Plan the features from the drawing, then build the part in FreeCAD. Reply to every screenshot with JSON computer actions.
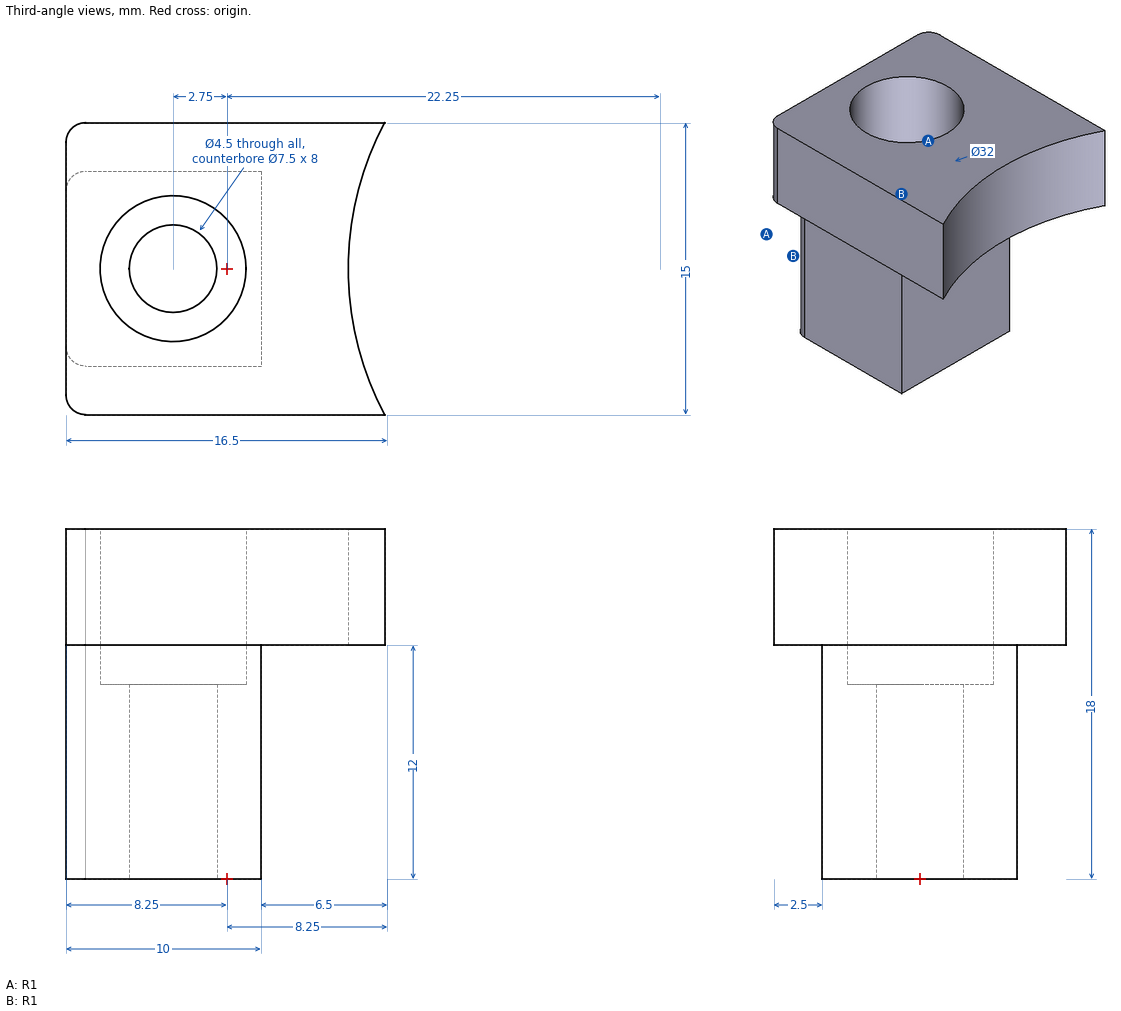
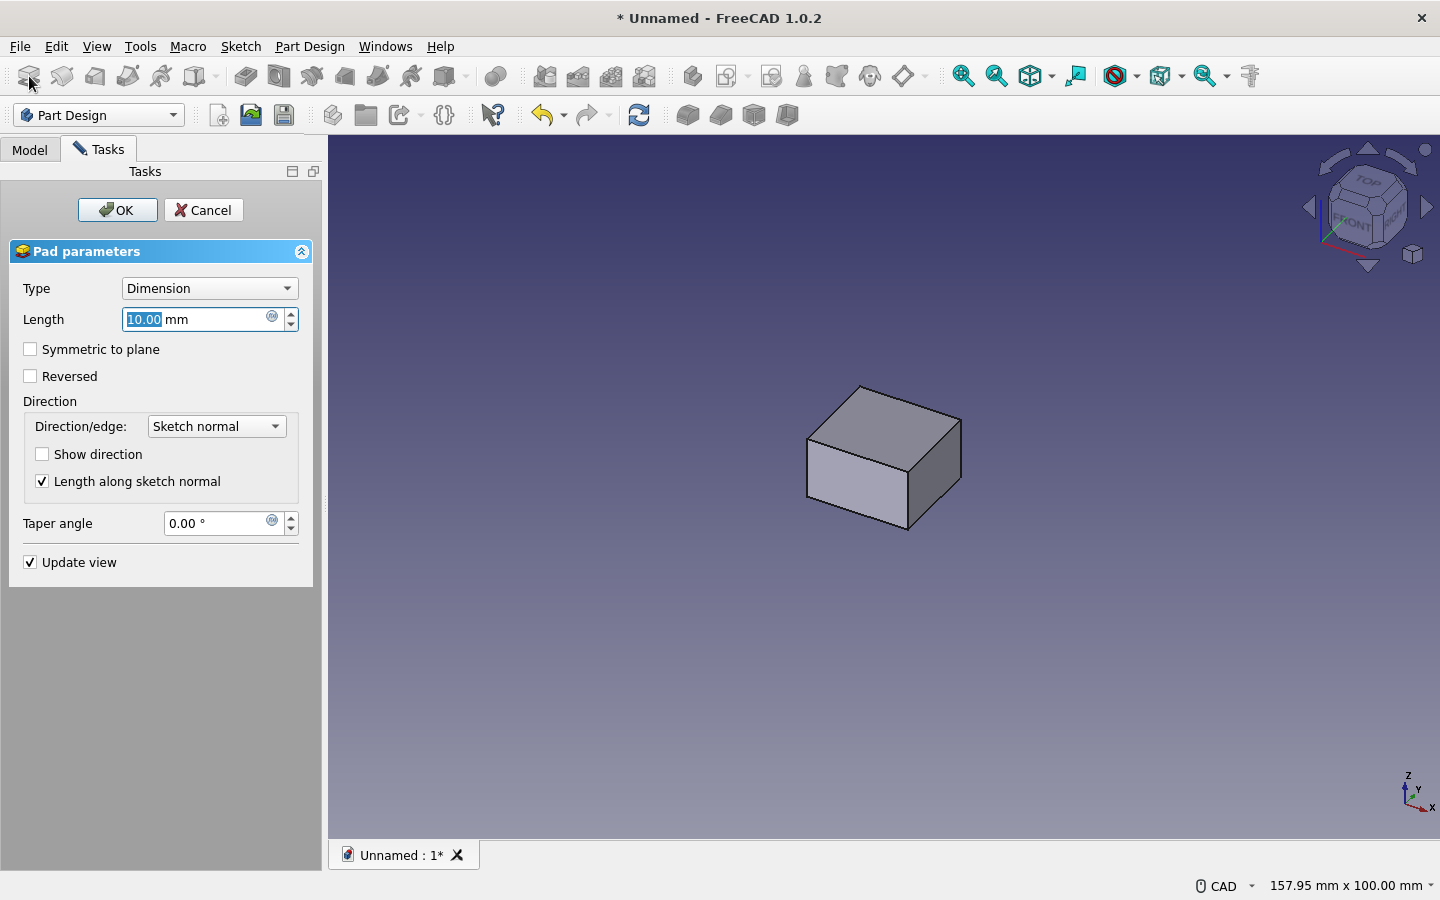
{"action": "type", "text": "18"}
{"action": "key", "text": "Tab"}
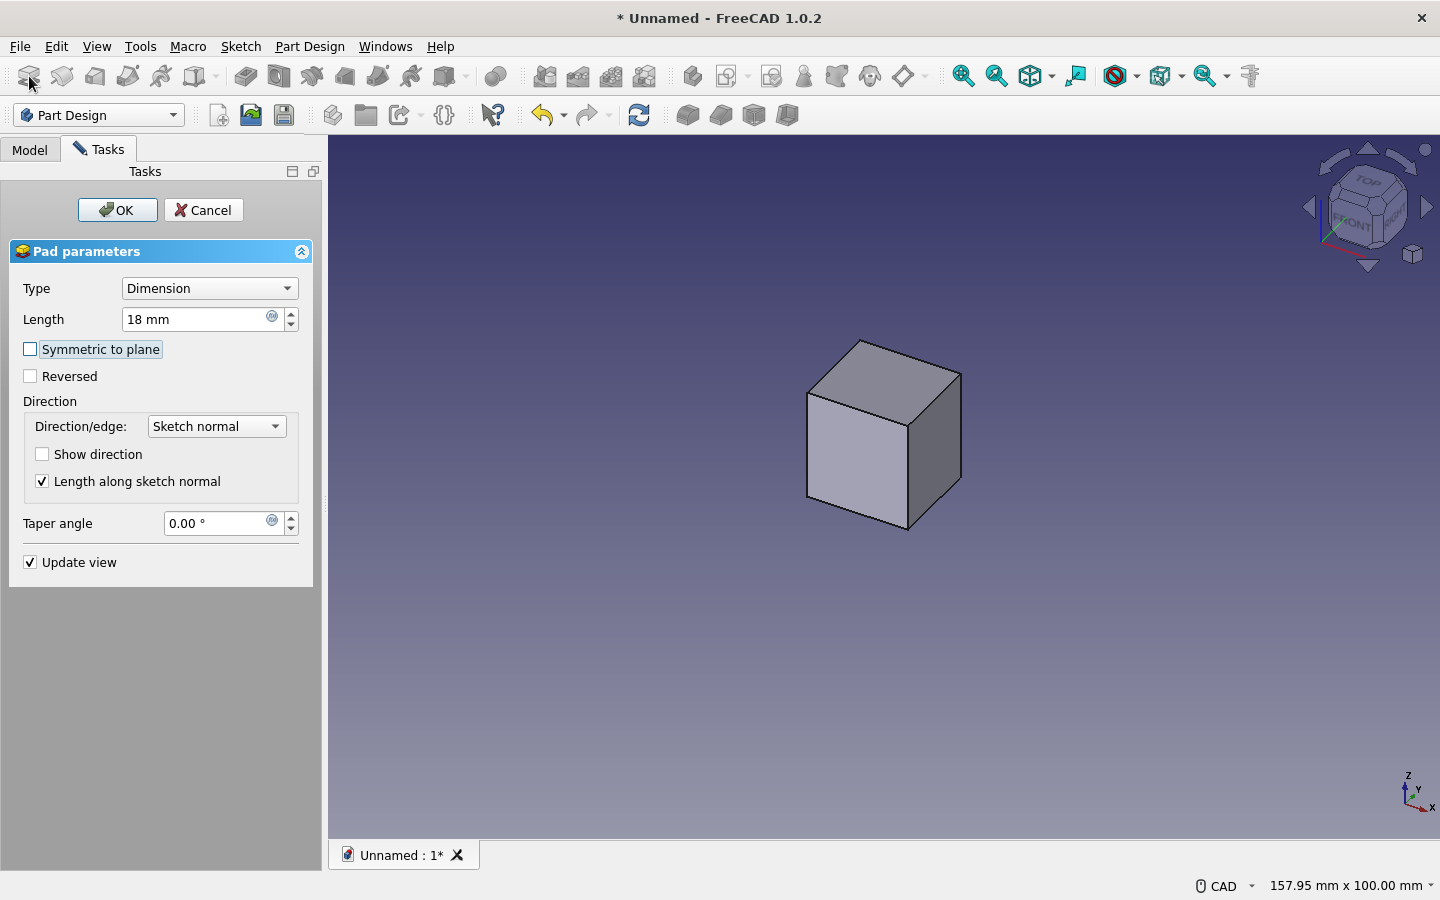
{"action": "left_click", "coordinate": [118, 210]}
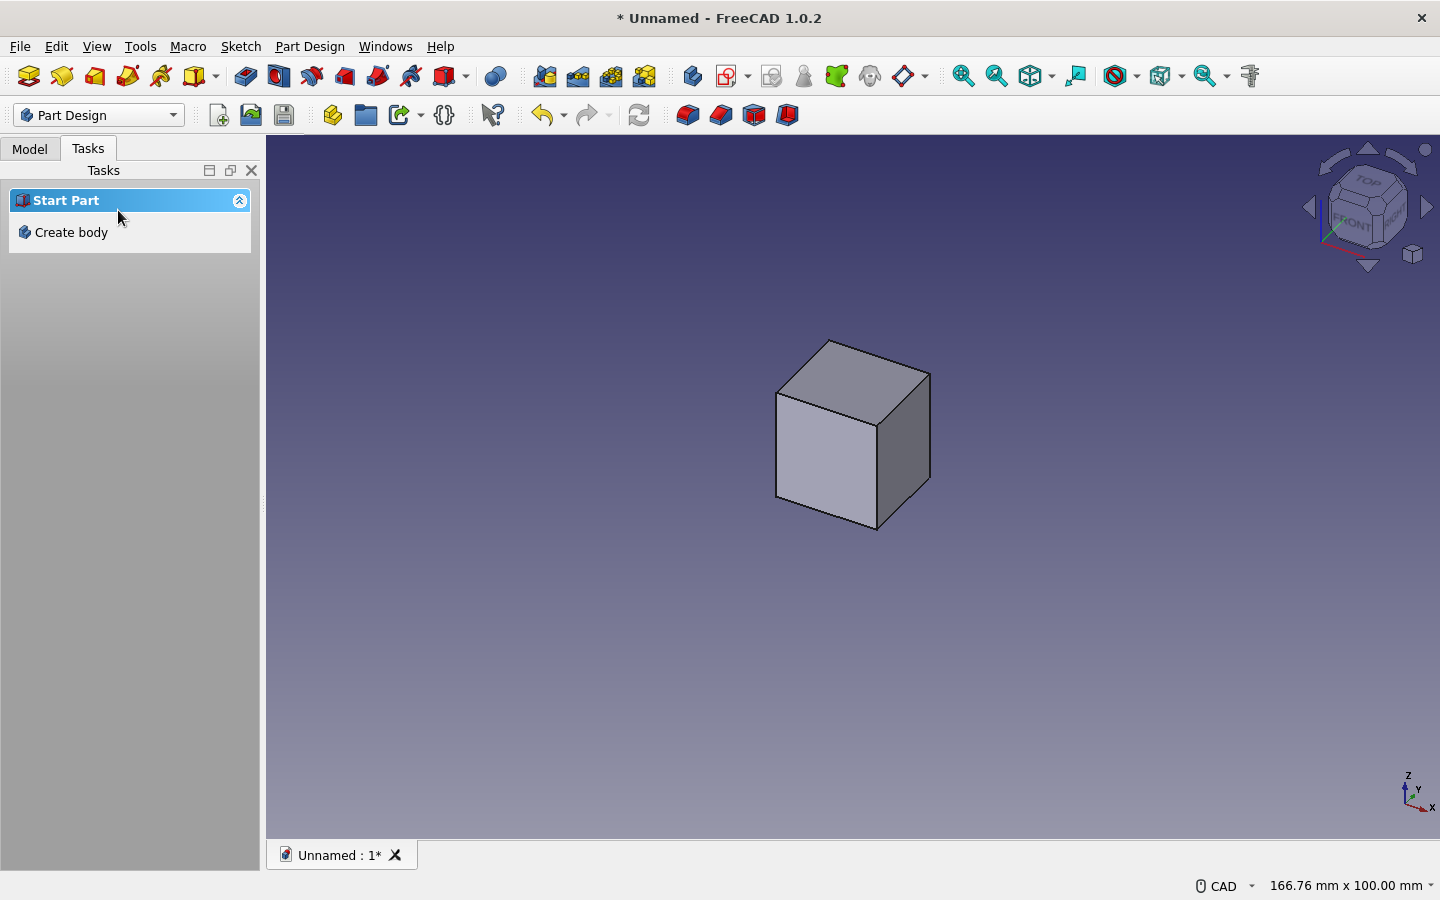
{"action": "left_click", "coordinate": [964, 76]}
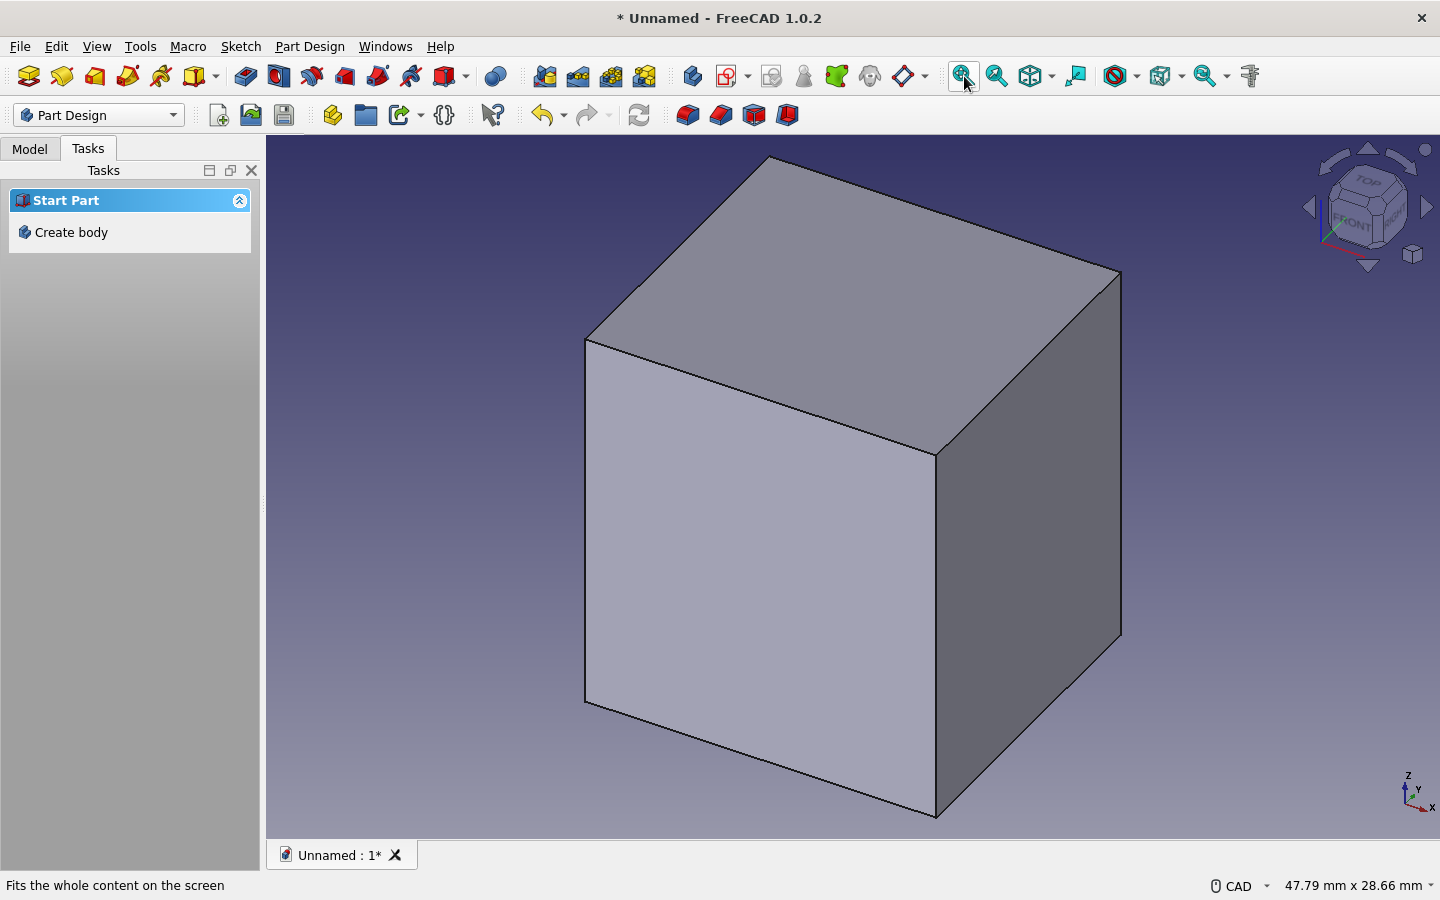
{"action": "key", "text": "0"}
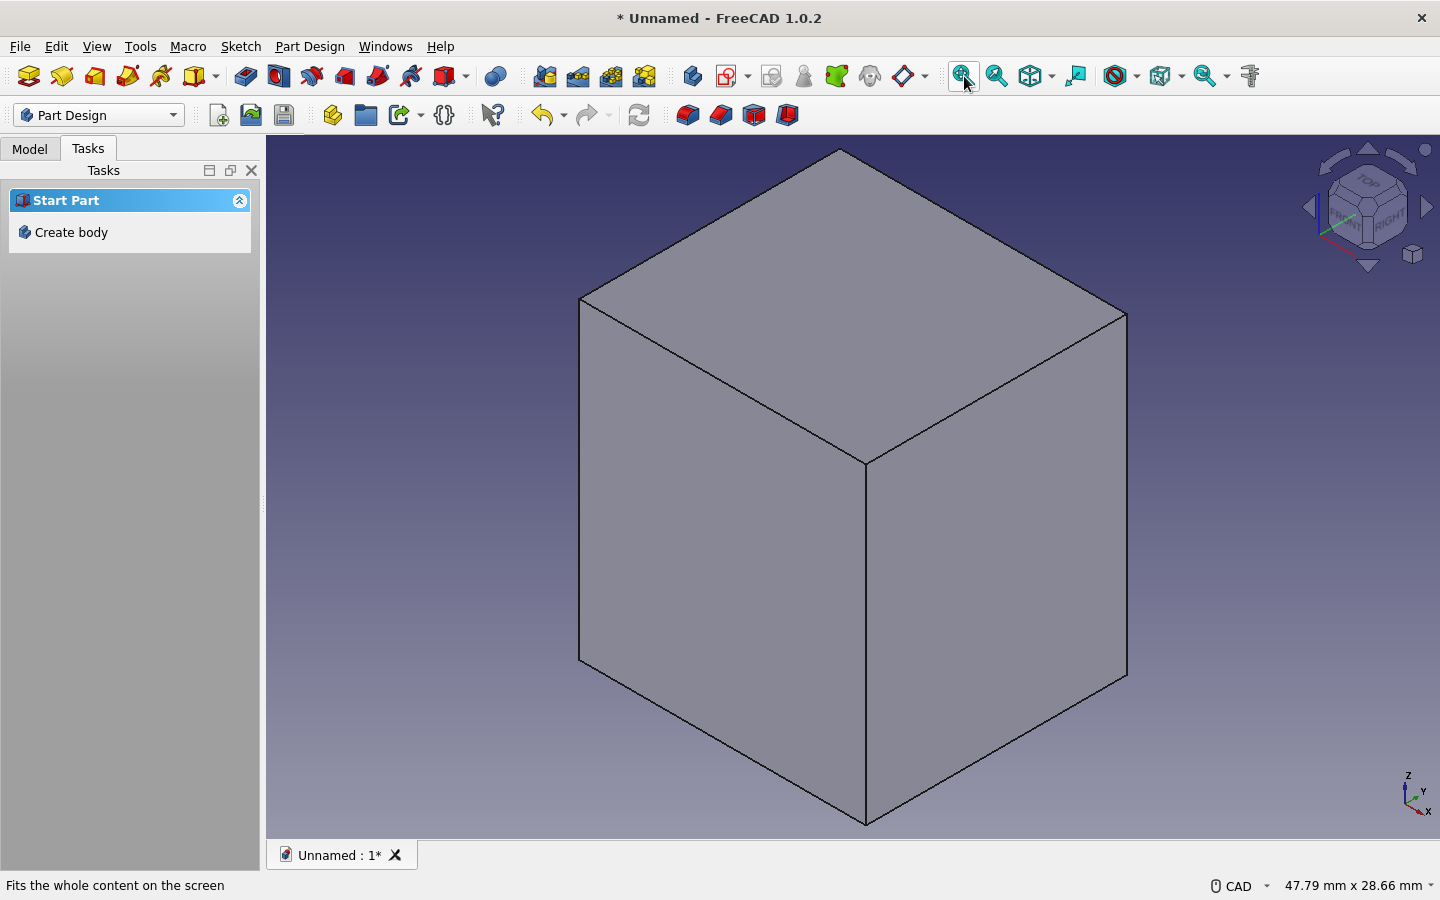
{"action": "key", "text": "2"}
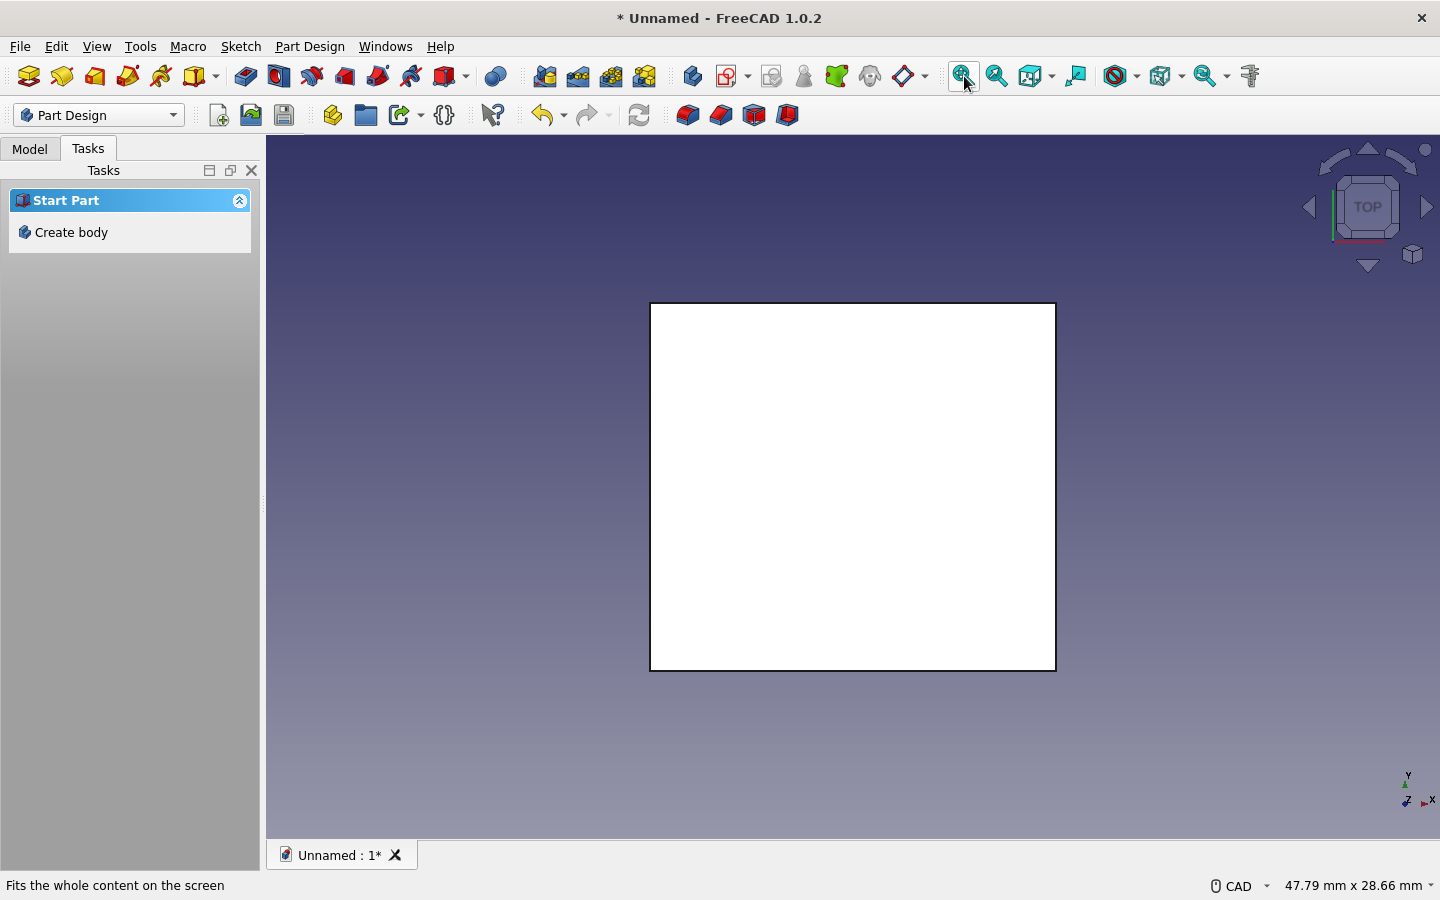
{"action": "key", "text": "1"}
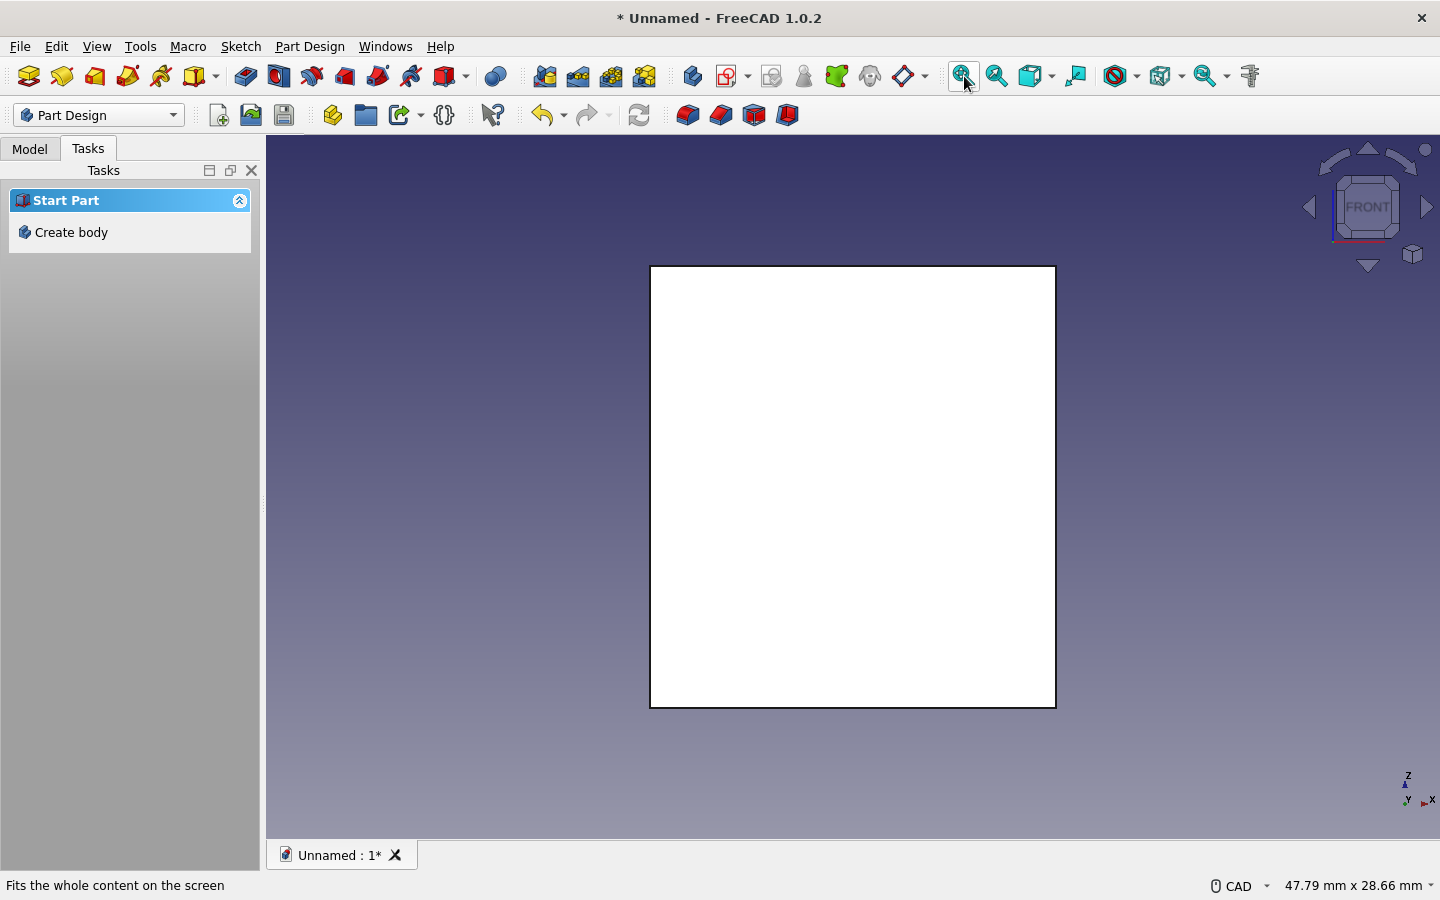
{"action": "left_click", "coordinate": [650, 486]}